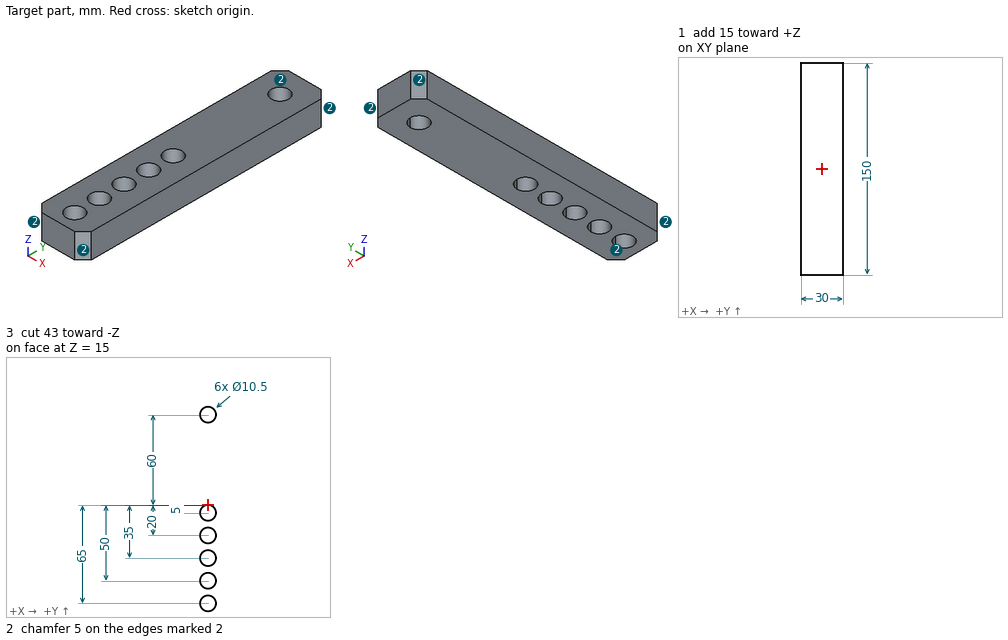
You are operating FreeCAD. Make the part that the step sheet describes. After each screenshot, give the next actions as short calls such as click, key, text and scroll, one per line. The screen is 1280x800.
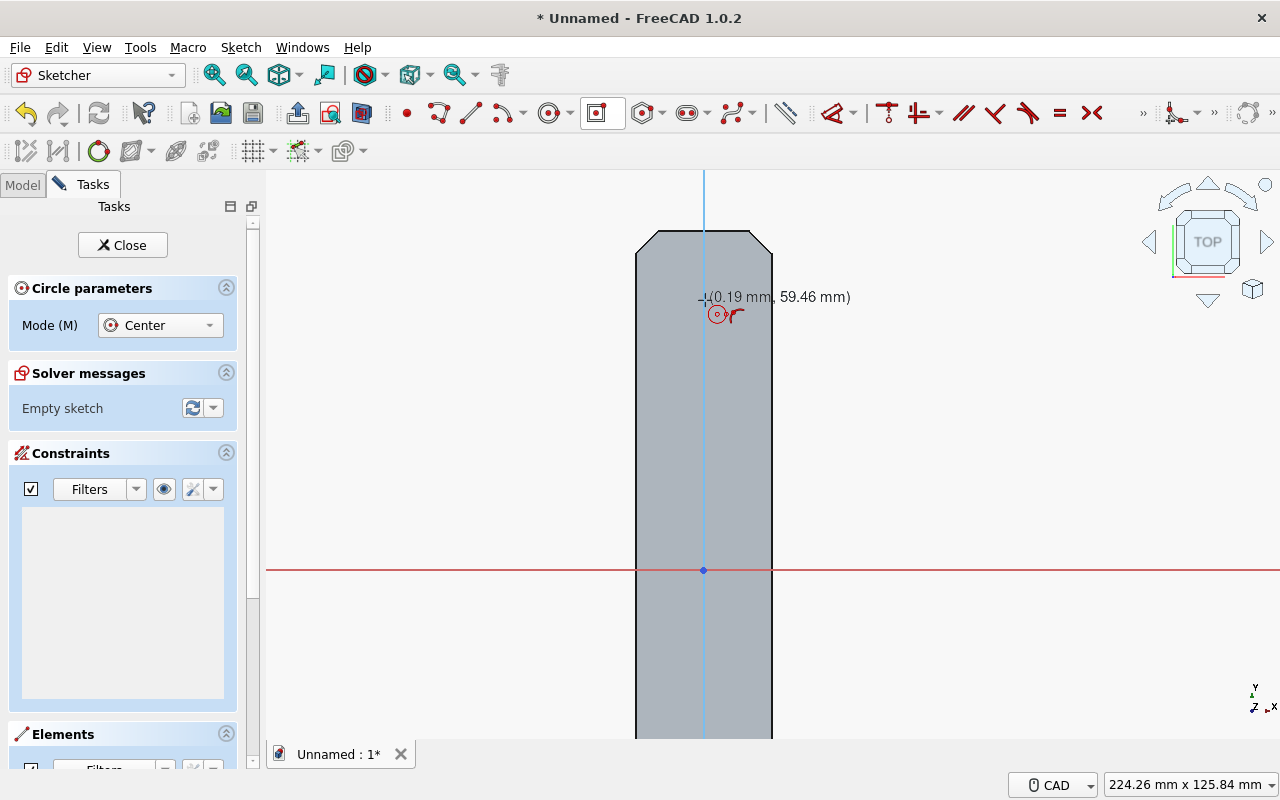
click(704, 299)
click(721, 282)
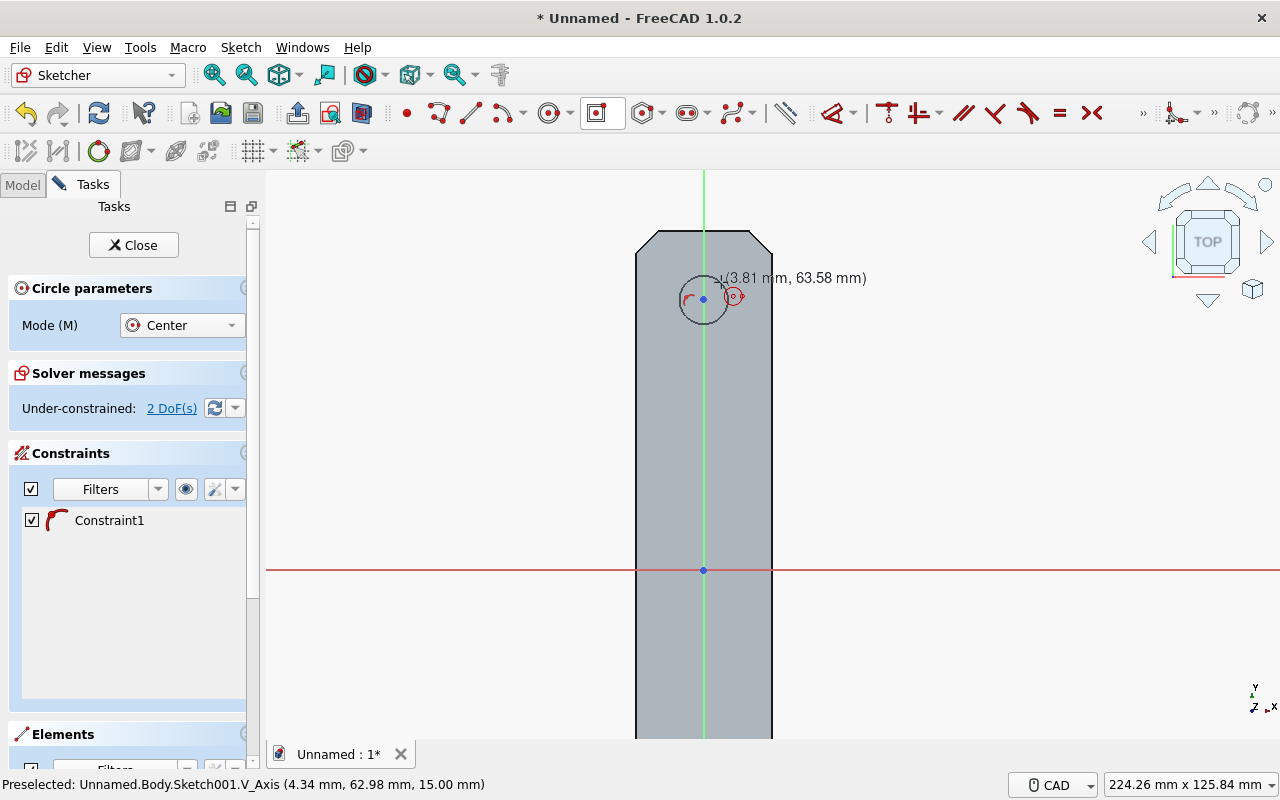
click(704, 593)
click(721, 610)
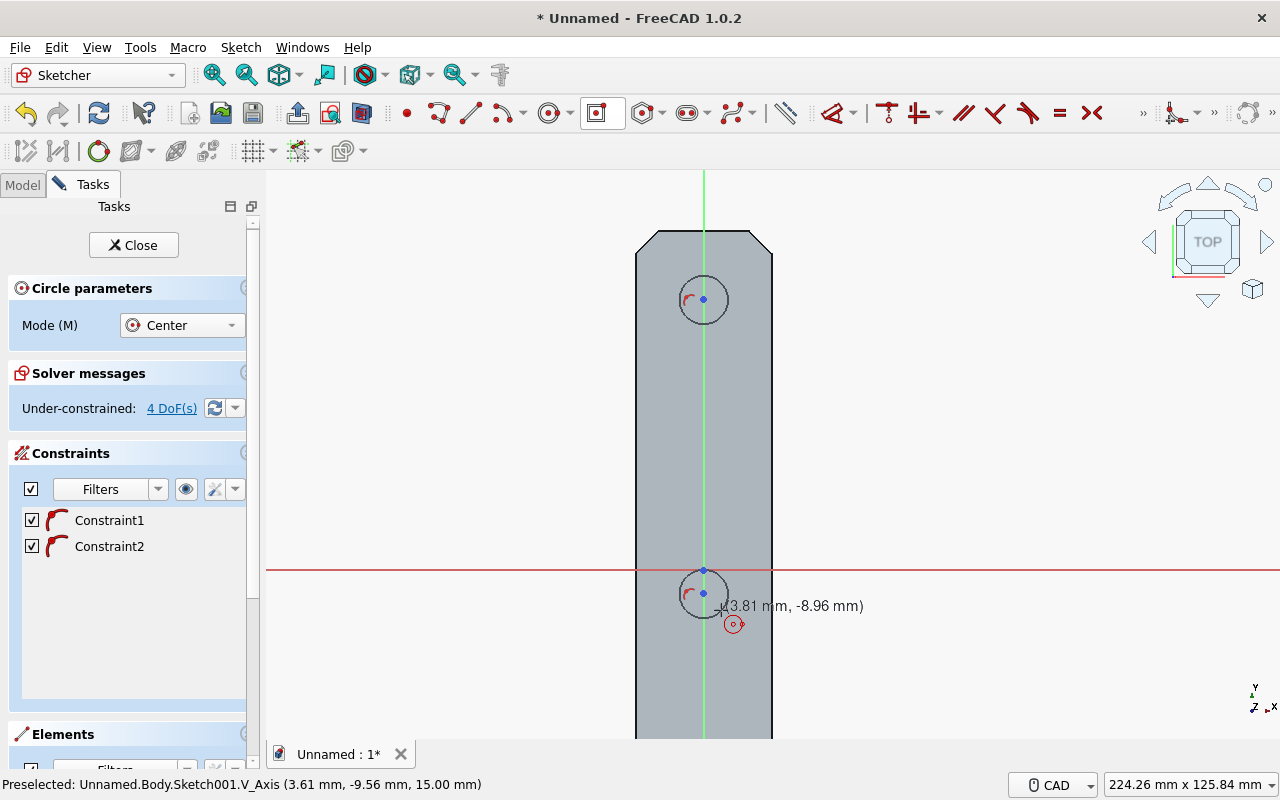
click(704, 661)
click(721, 644)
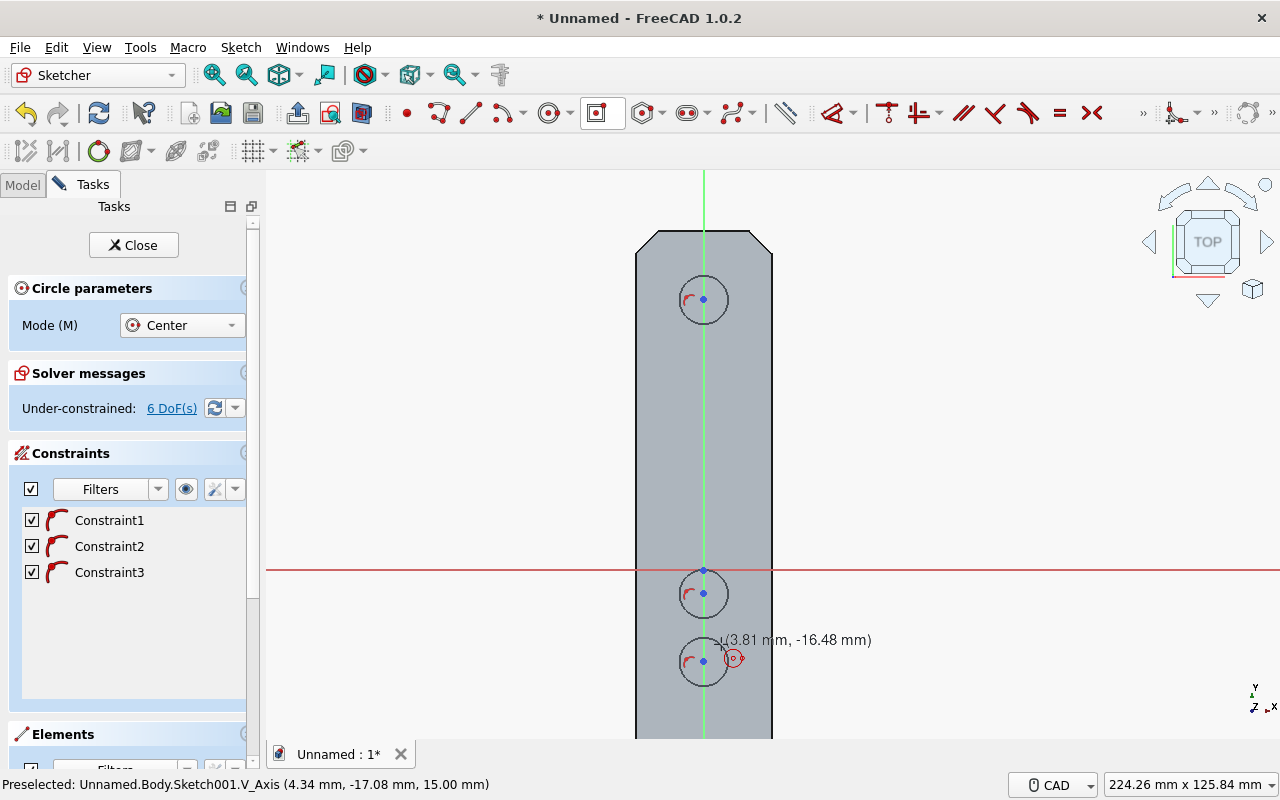
scroll(705, 300, down, 3)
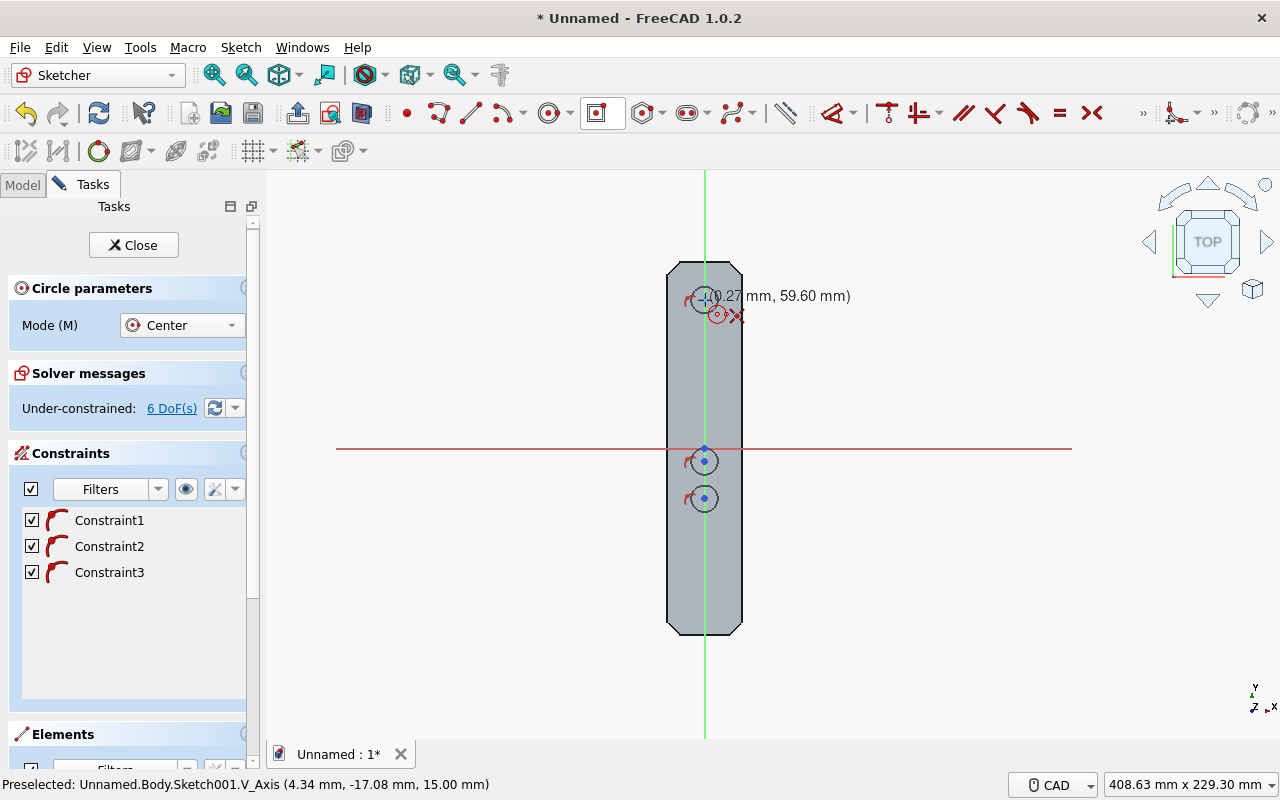
scroll(705, 535, up, 3)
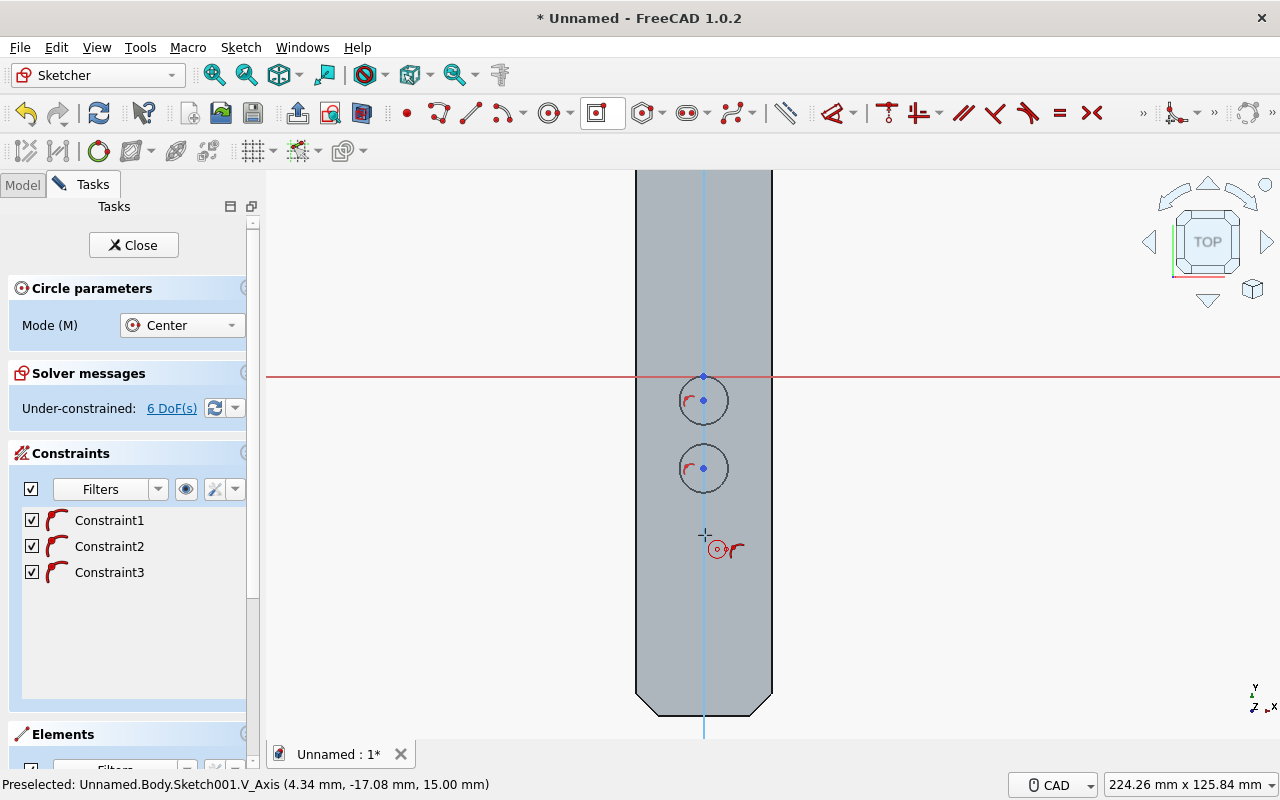
click(704, 535)
click(721, 518)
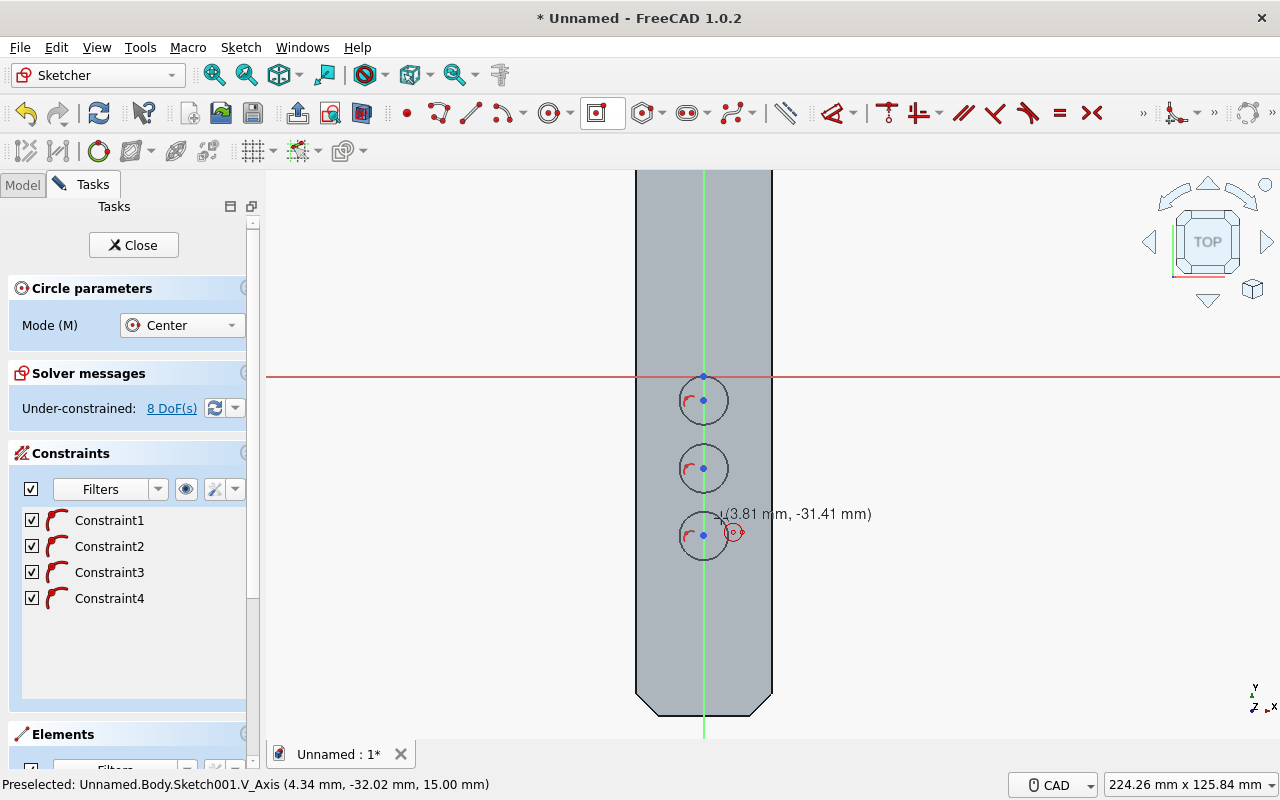
click(704, 603)
click(721, 586)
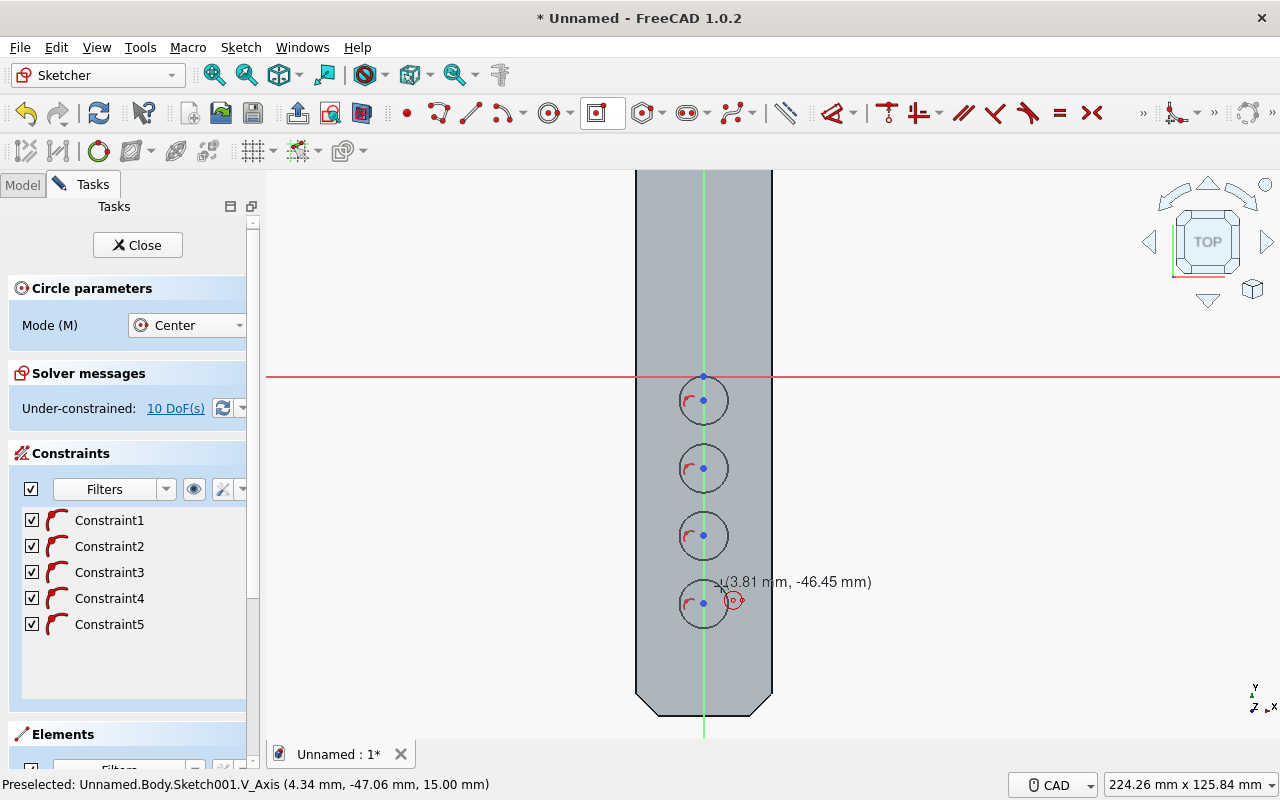
click(704, 671)
click(721, 654)
key(Escape)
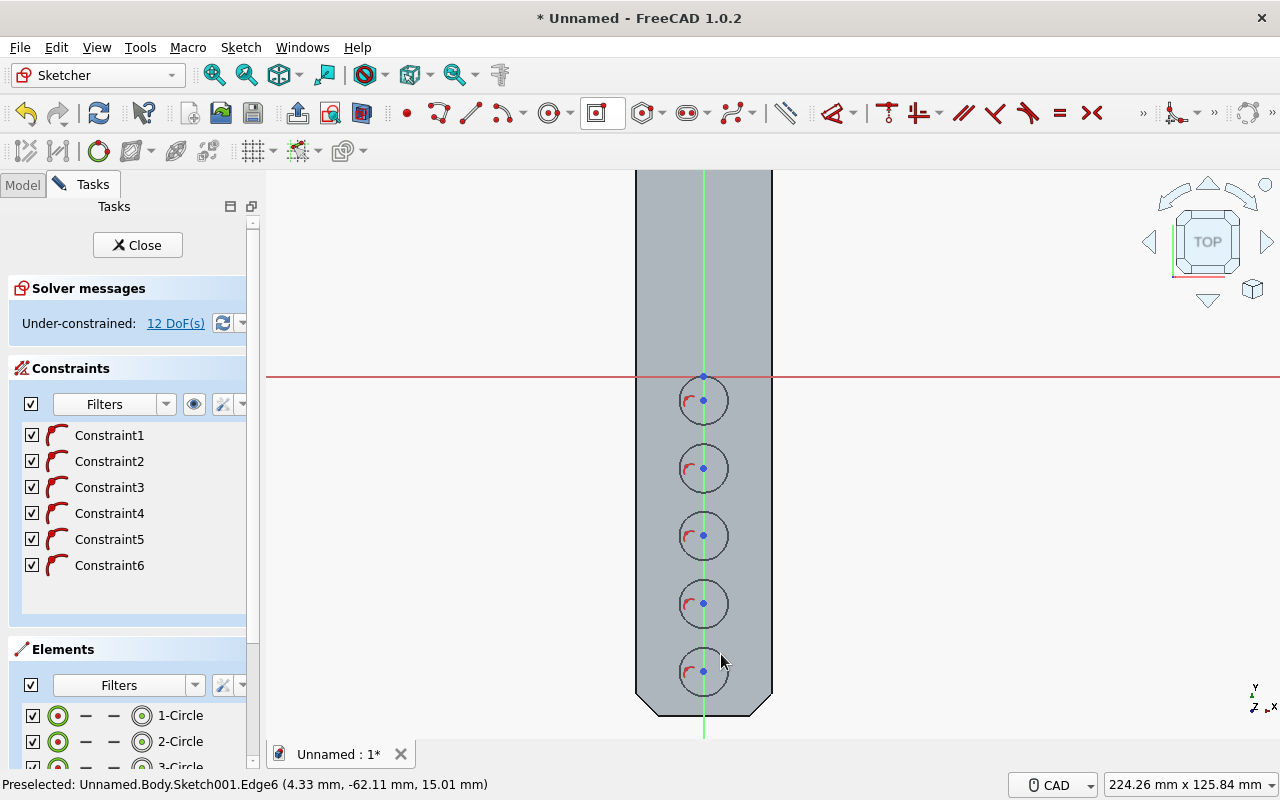
scroll(705, 535, down, 3)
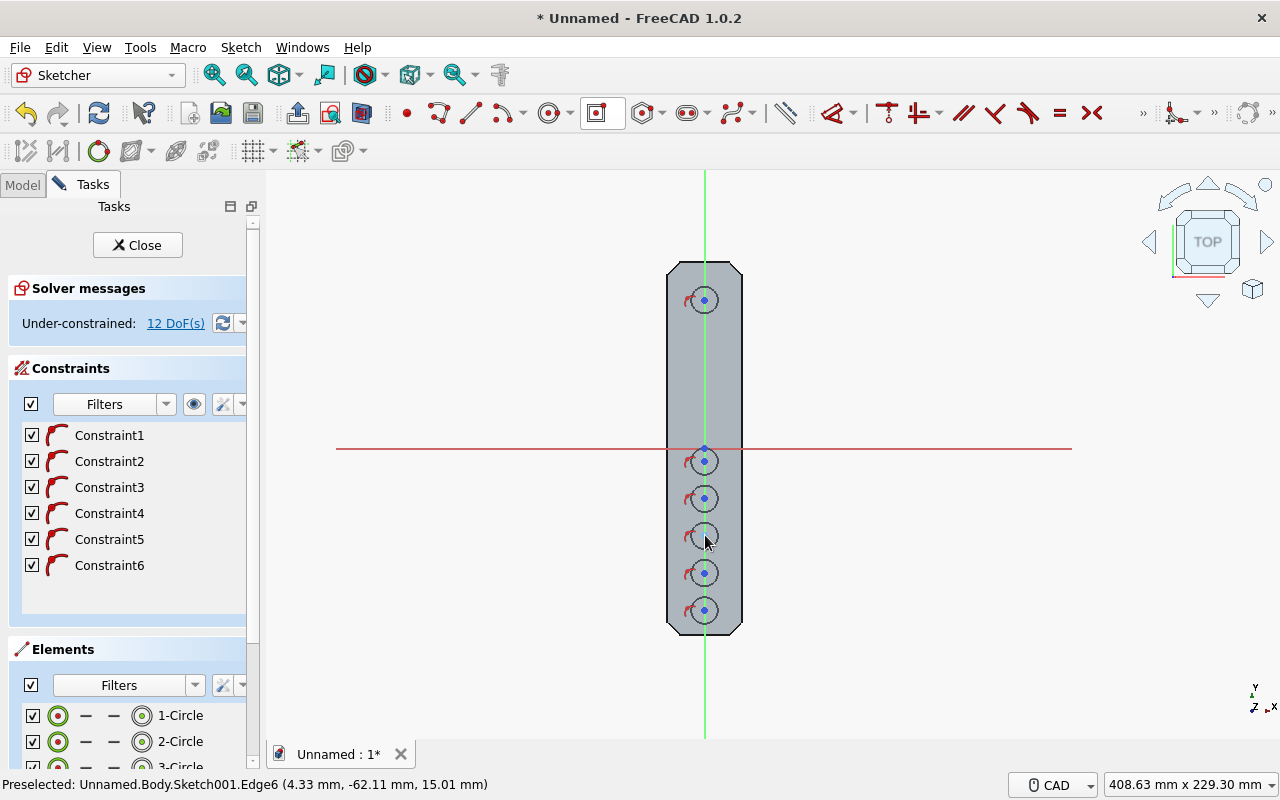
scroll(714, 291, up, 2)